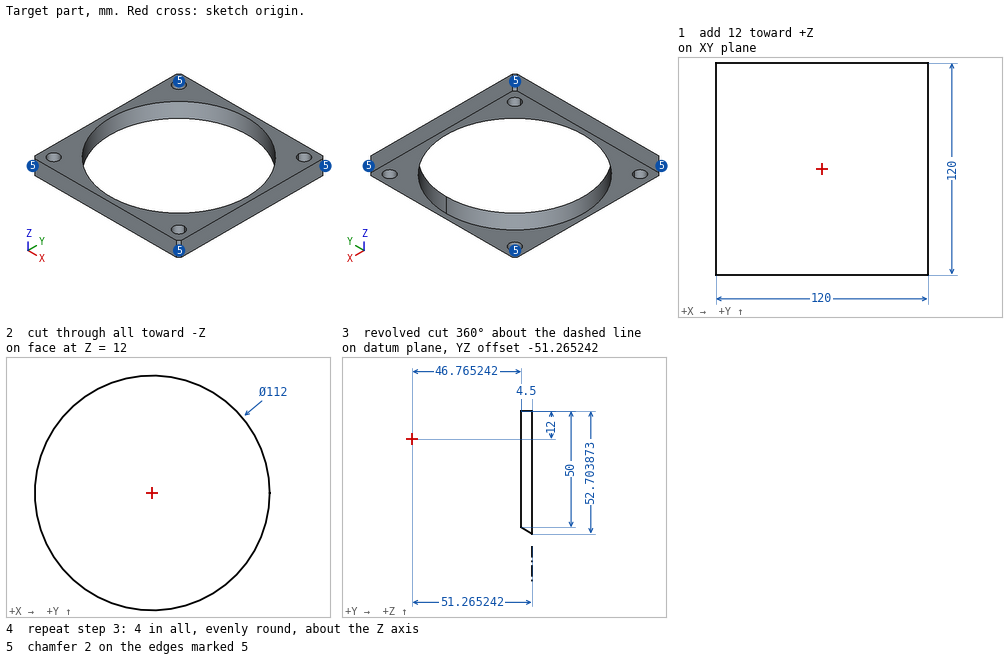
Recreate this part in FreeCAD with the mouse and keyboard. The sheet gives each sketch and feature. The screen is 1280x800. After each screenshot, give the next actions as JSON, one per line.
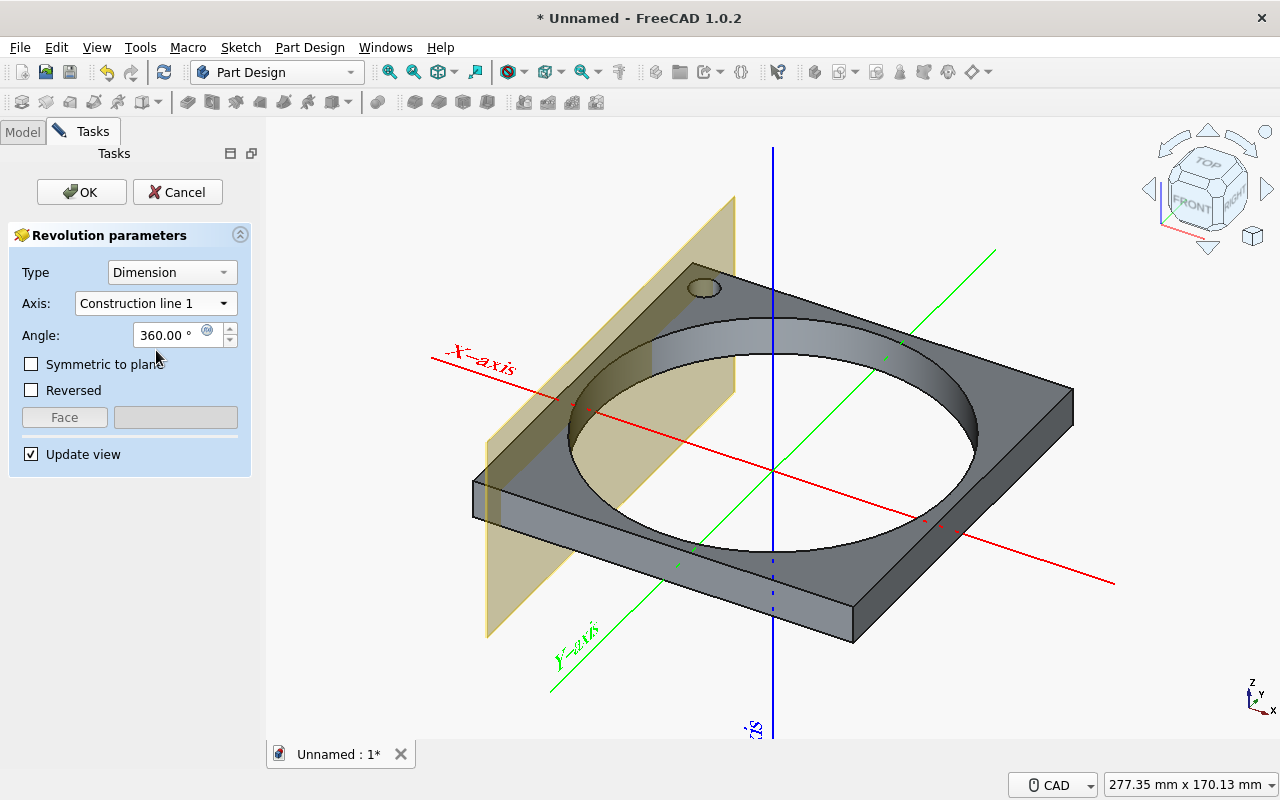
{"action": "left_click", "coordinate": [82, 192]}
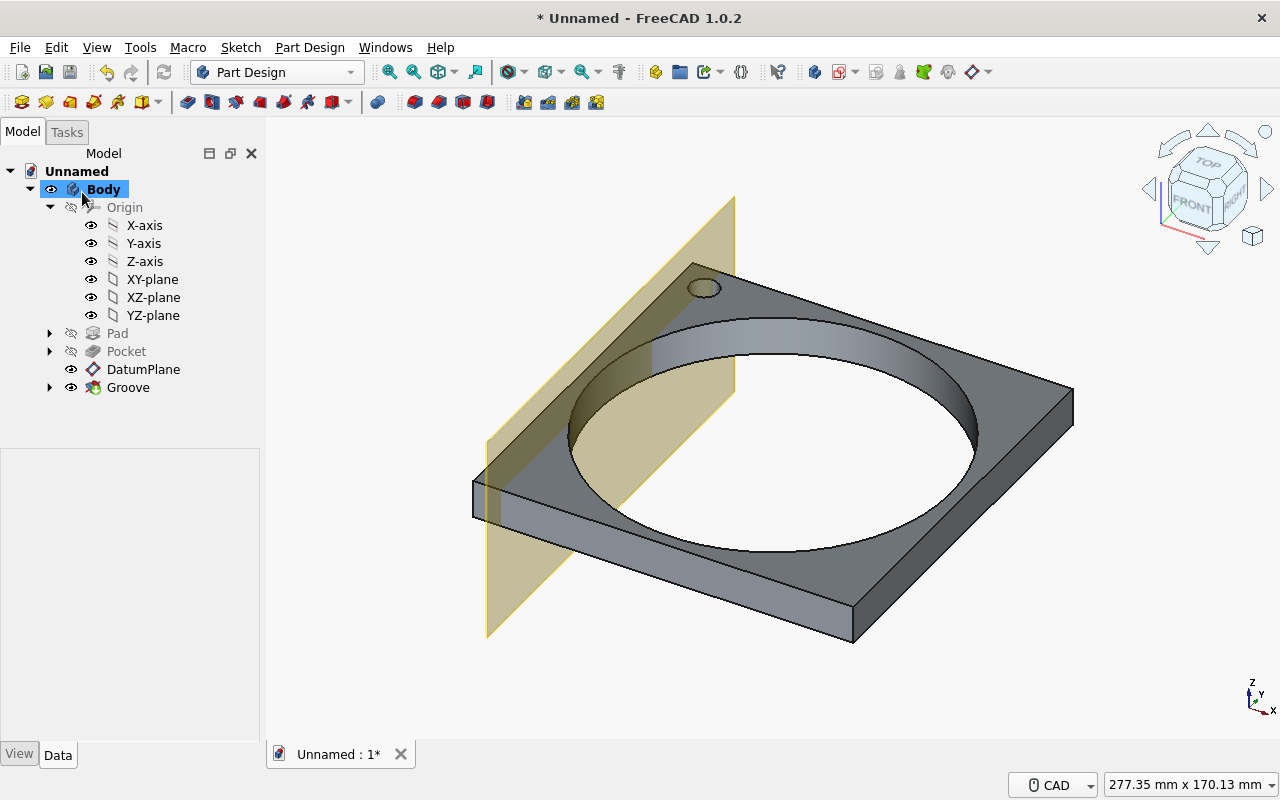
{"action": "left_click", "coordinate": [116, 369]}
{"action": "key", "text": "space"}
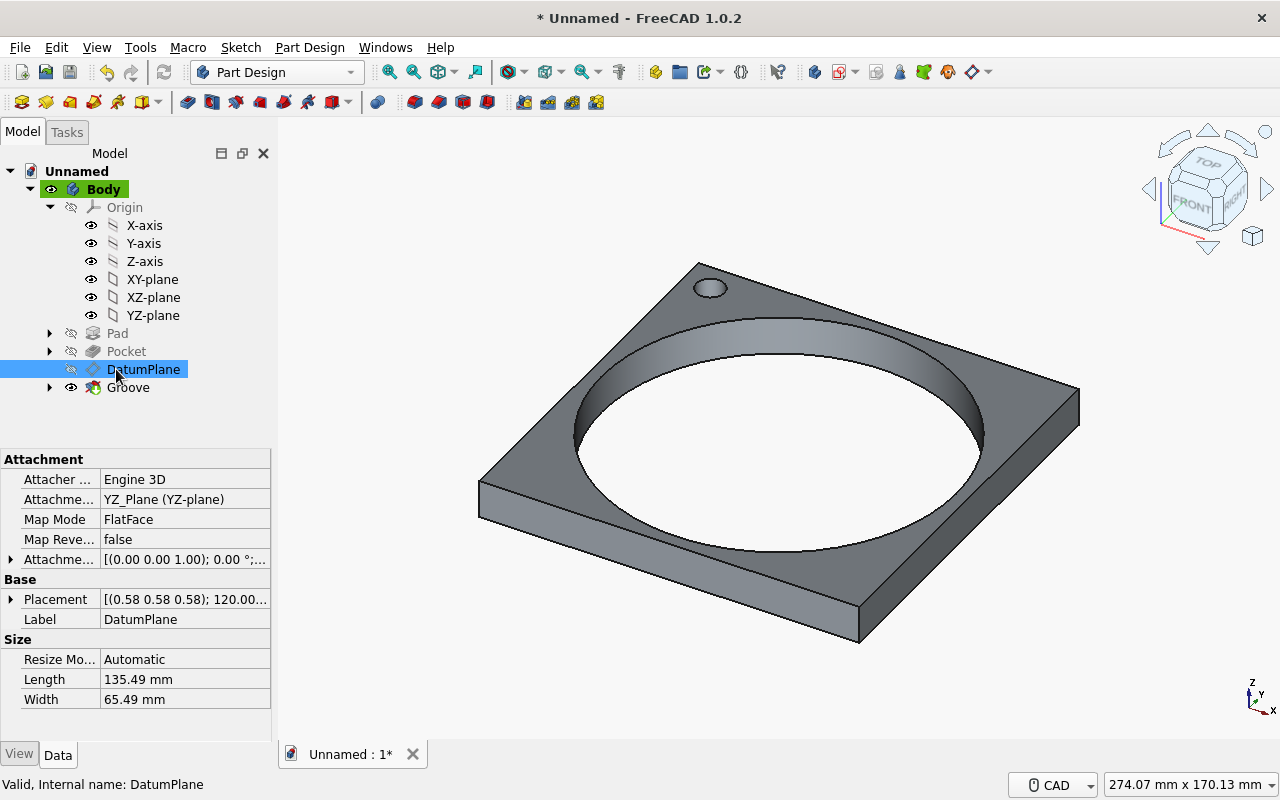
{"action": "left_click", "coordinate": [116, 387]}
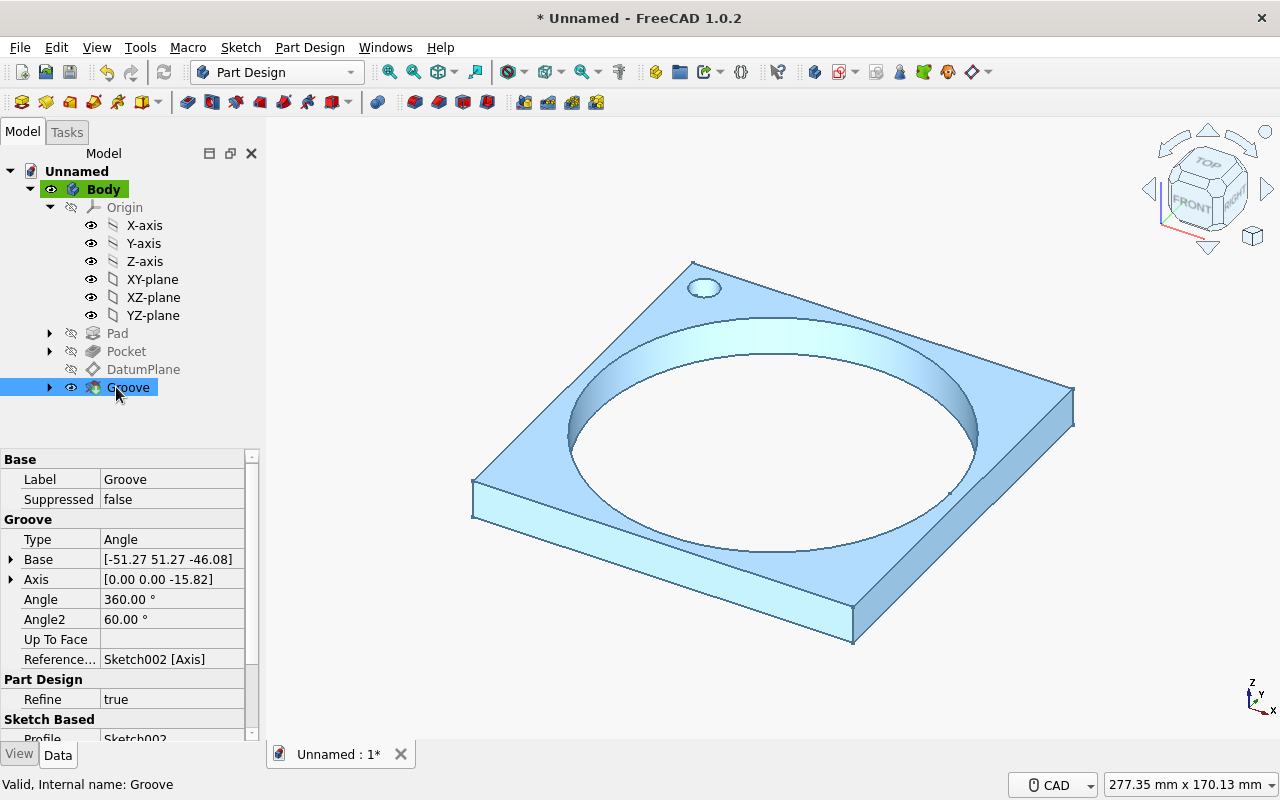
{"action": "left_click", "coordinate": [572, 102]}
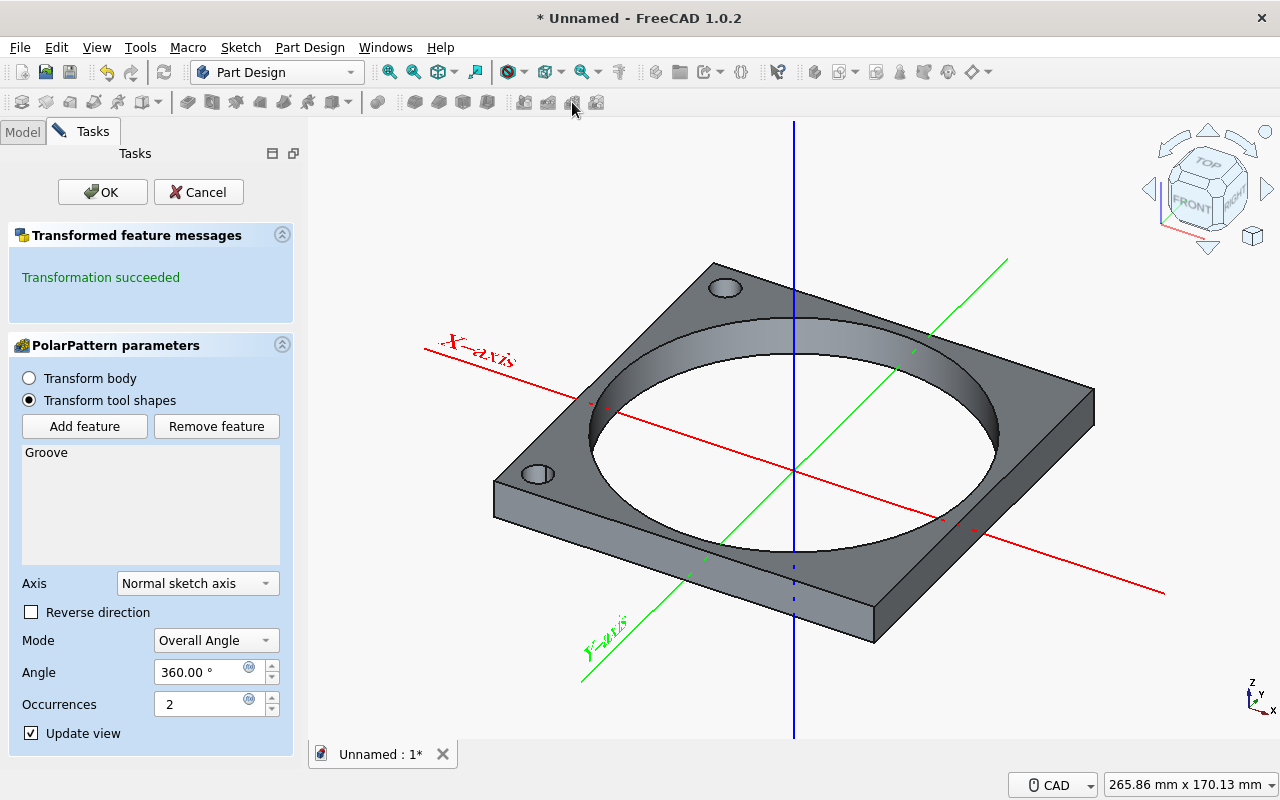
{"action": "left_click", "coordinate": [198, 584]}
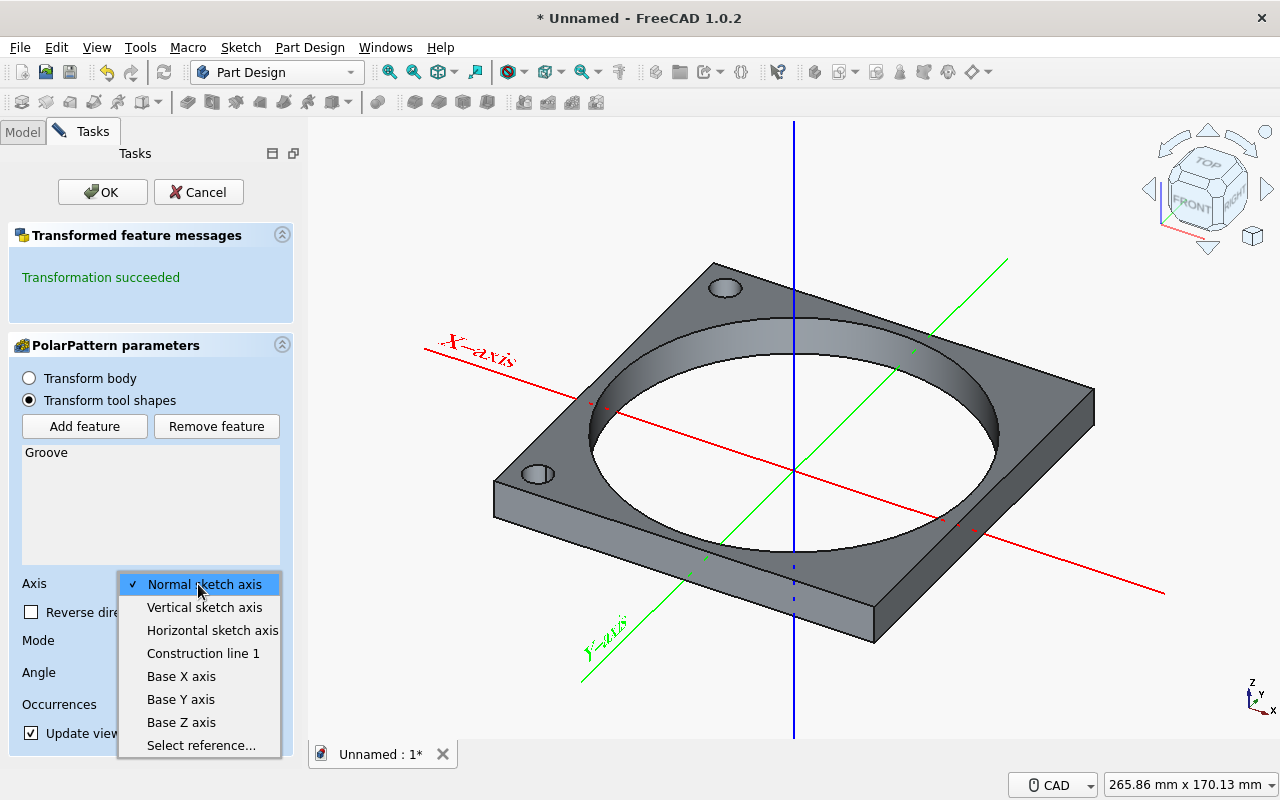
{"action": "left_click", "coordinate": [198, 722]}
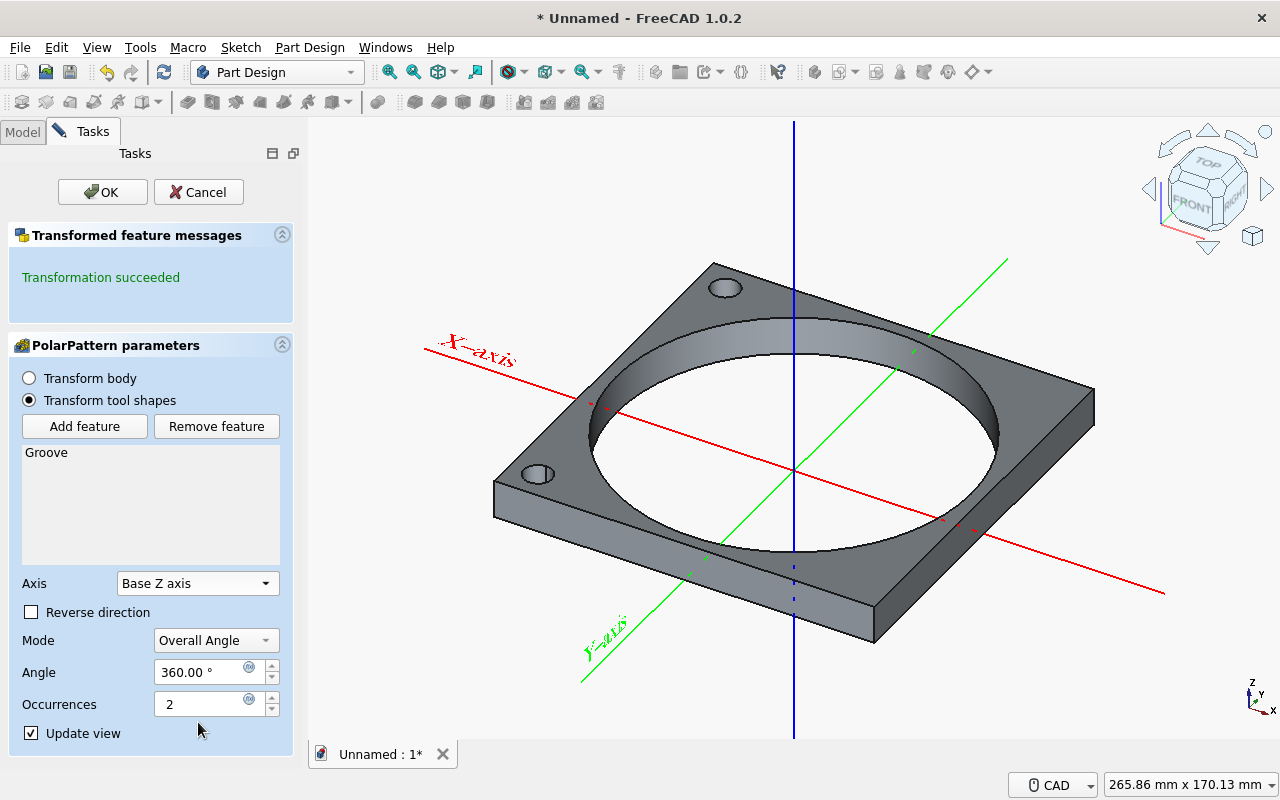
{"action": "triple_click", "coordinate": [209, 704]}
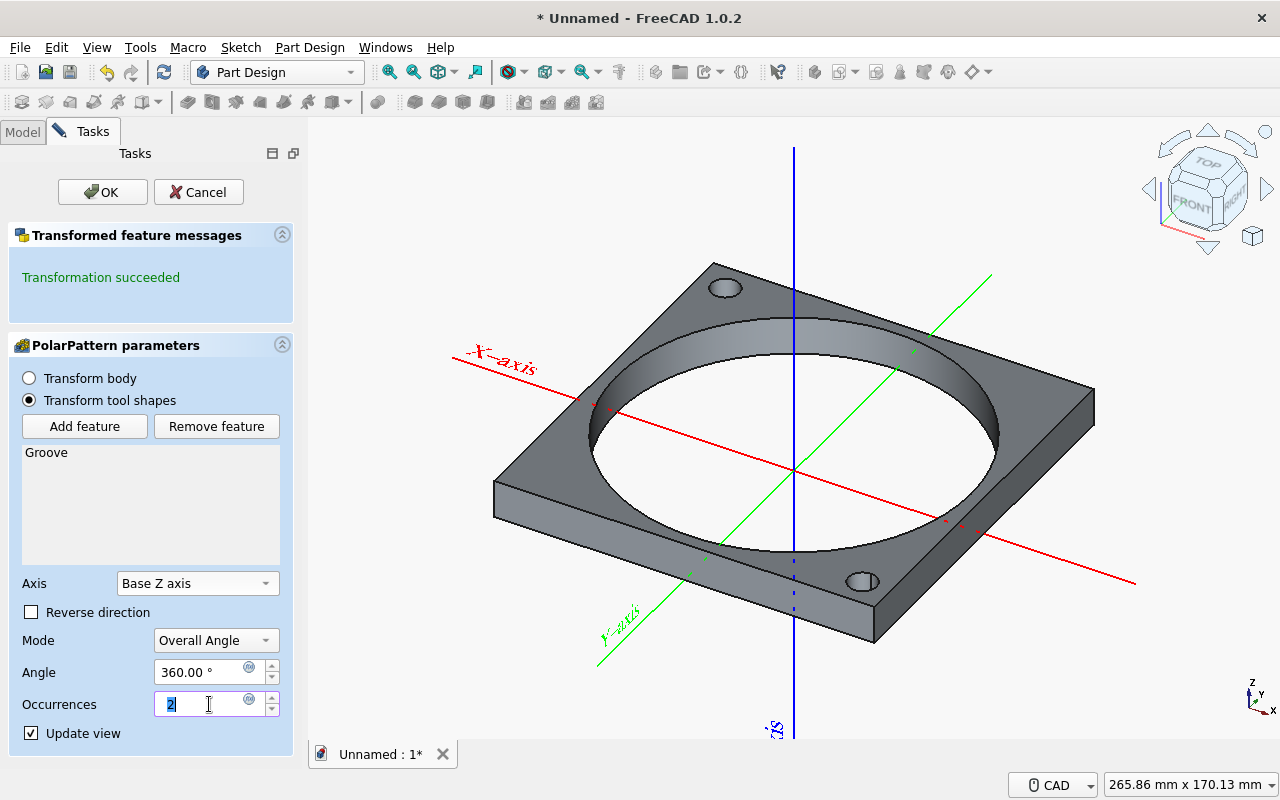
{"action": "type", "text": "4"}
{"action": "key", "text": "Tab"}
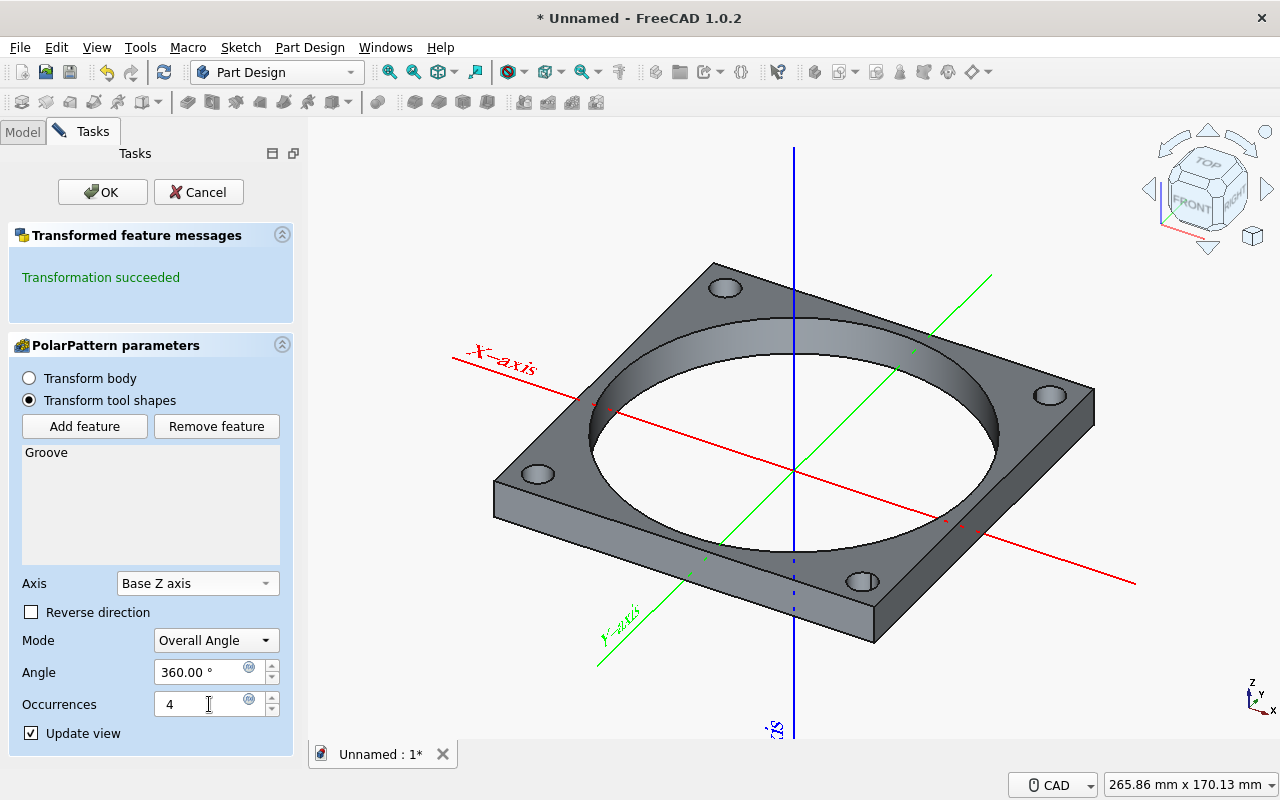
{"action": "left_click", "coordinate": [103, 192]}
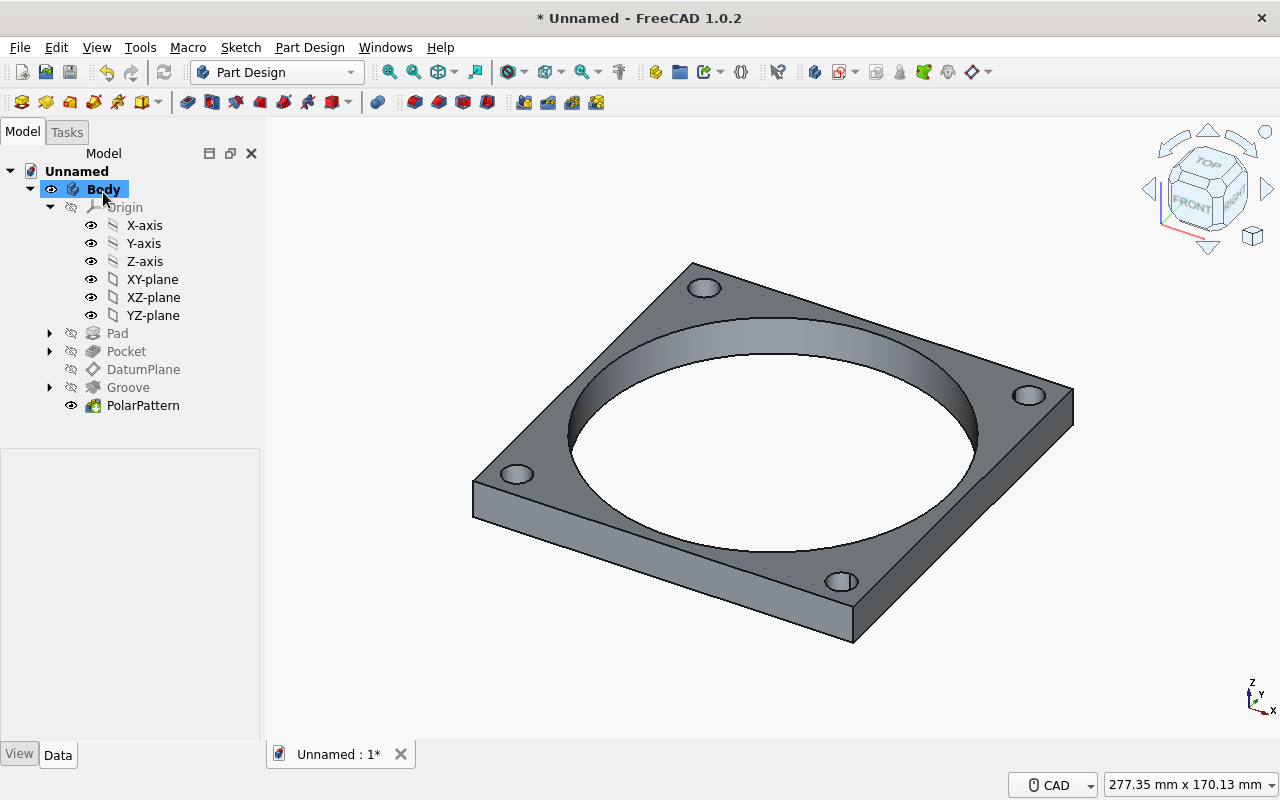
{"action": "left_click", "coordinate": [853, 624]}